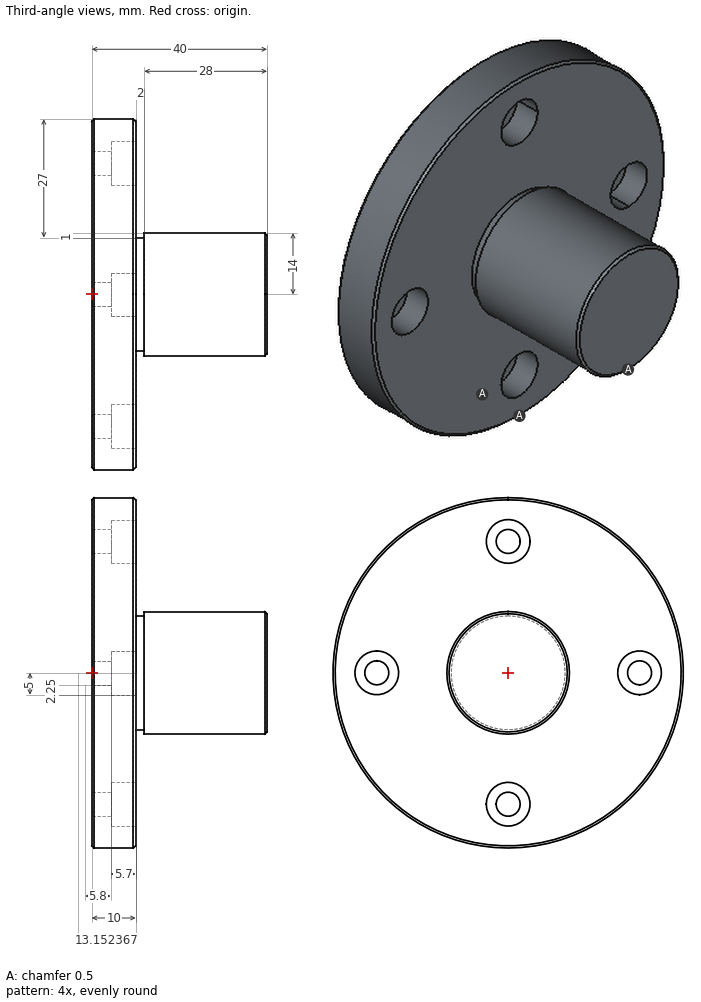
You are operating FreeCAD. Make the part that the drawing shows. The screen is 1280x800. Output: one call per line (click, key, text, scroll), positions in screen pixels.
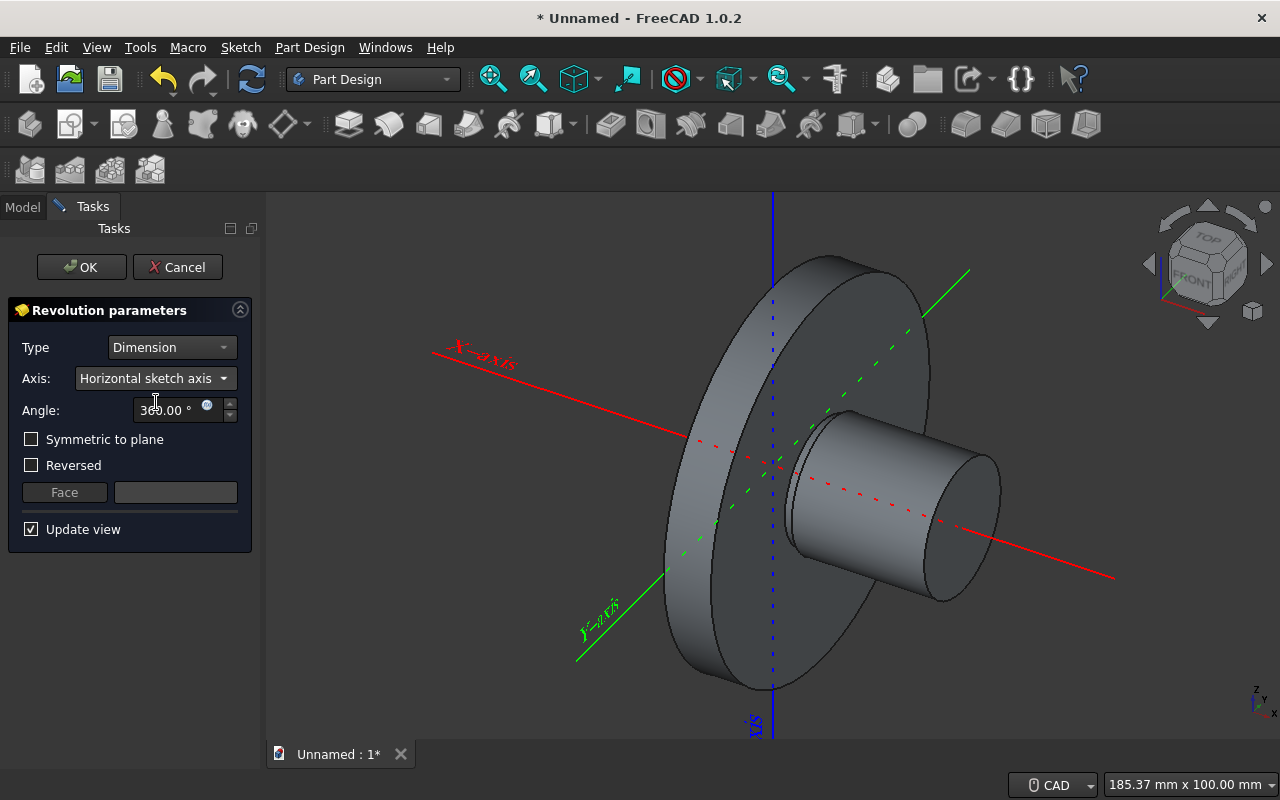
click(82, 267)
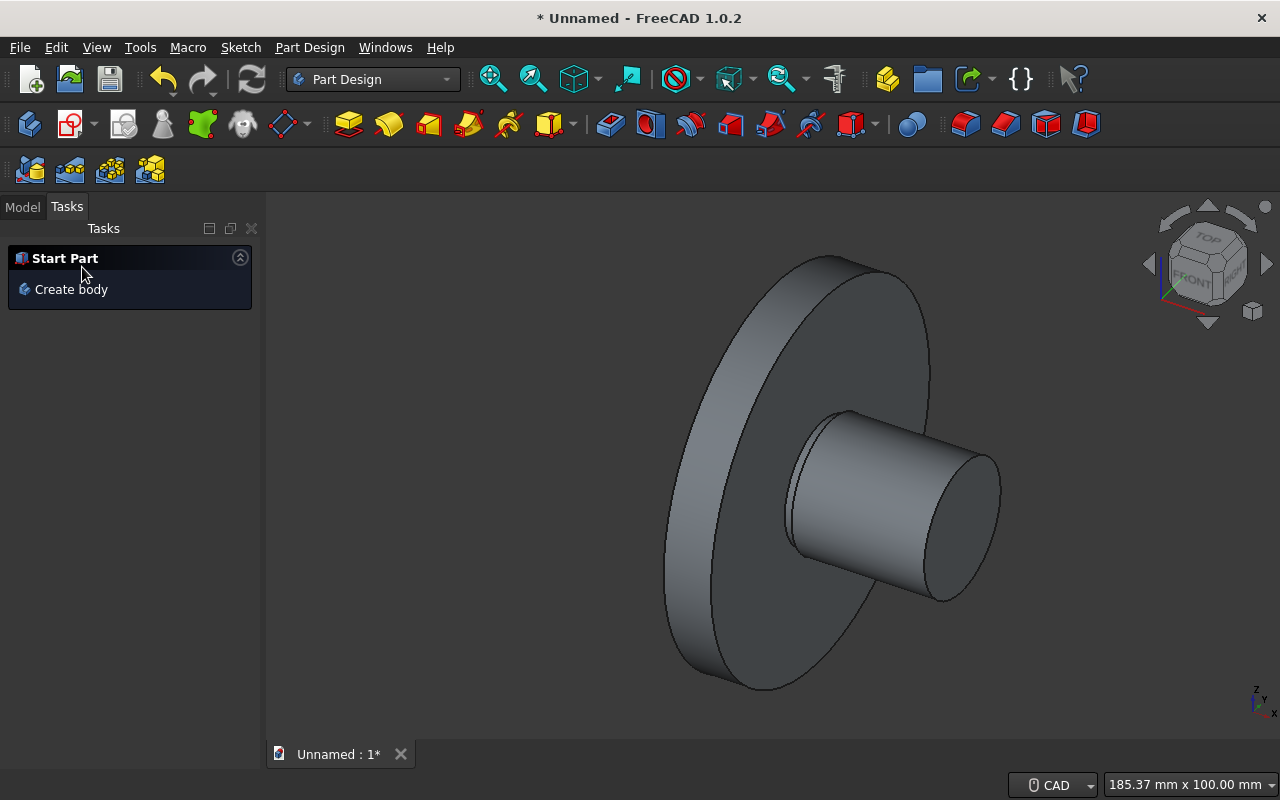
click(494, 80)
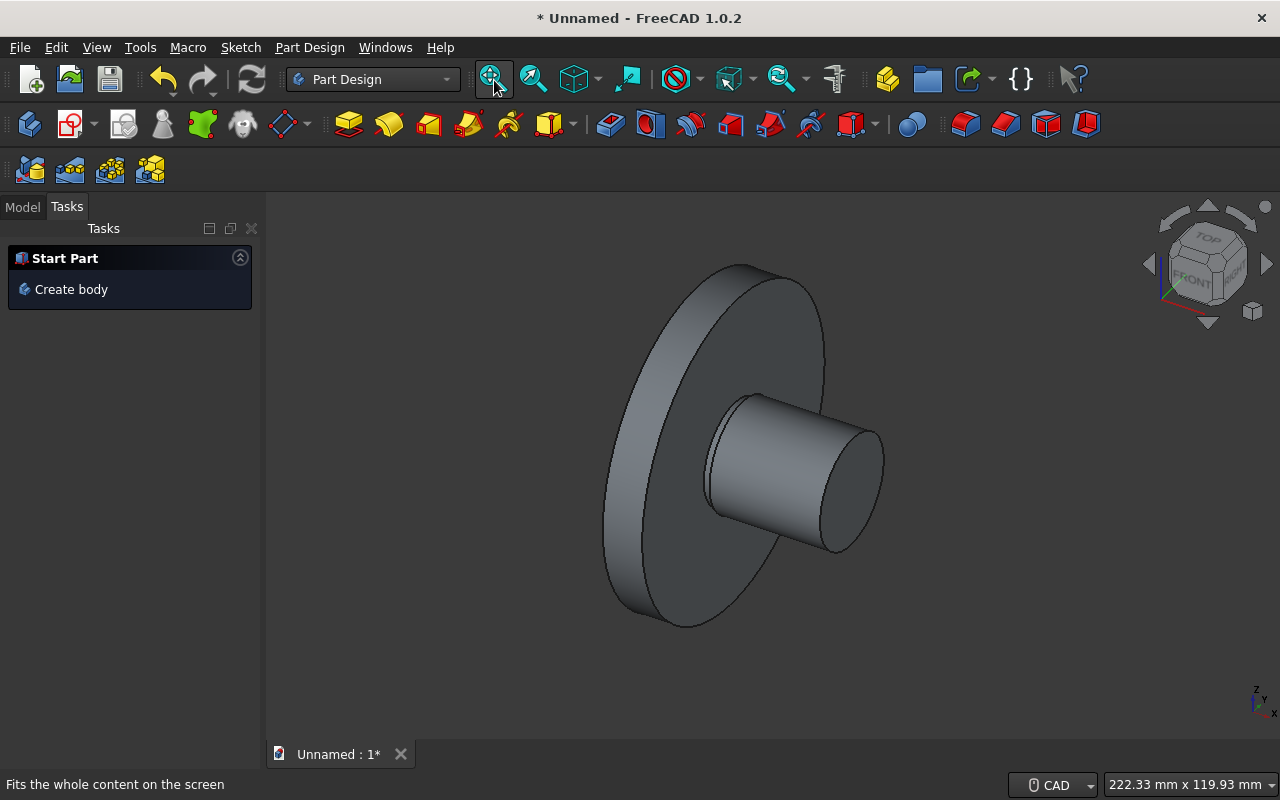
click(820, 522)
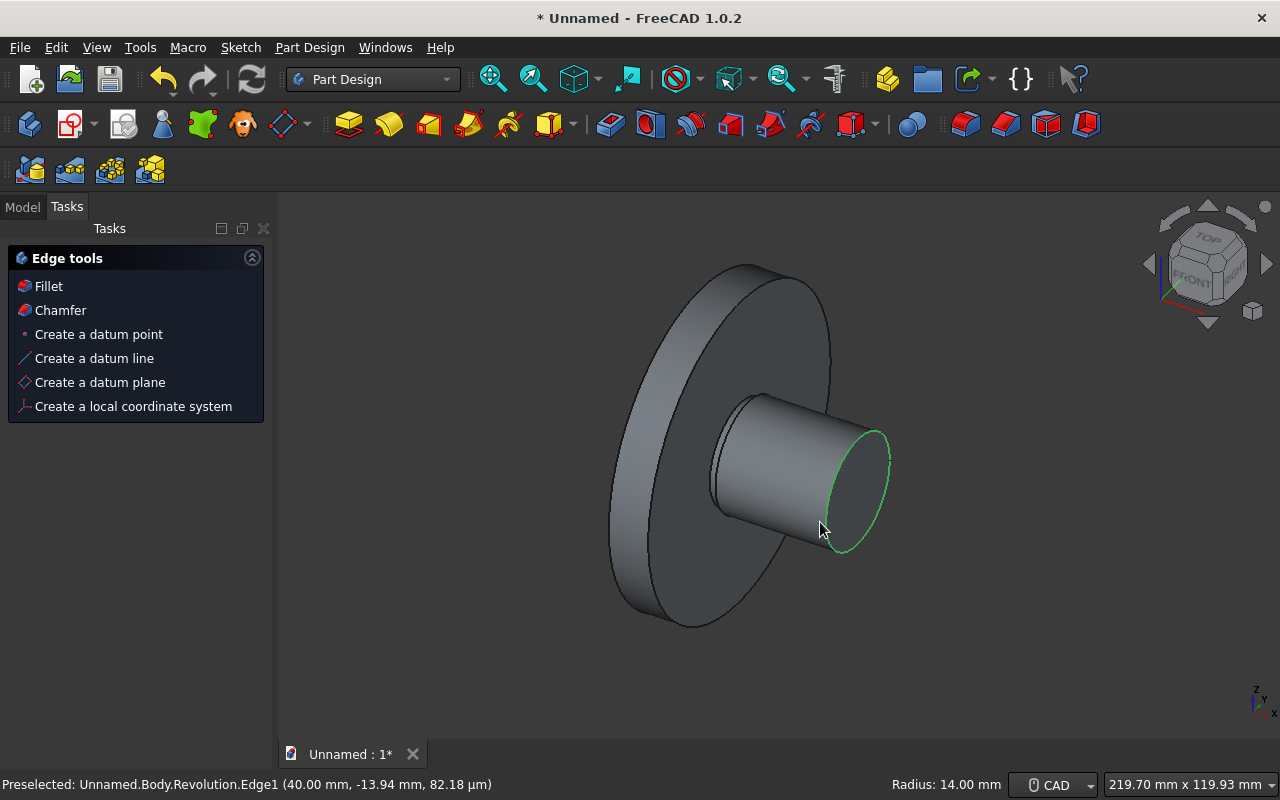
click(648, 542, ctrl)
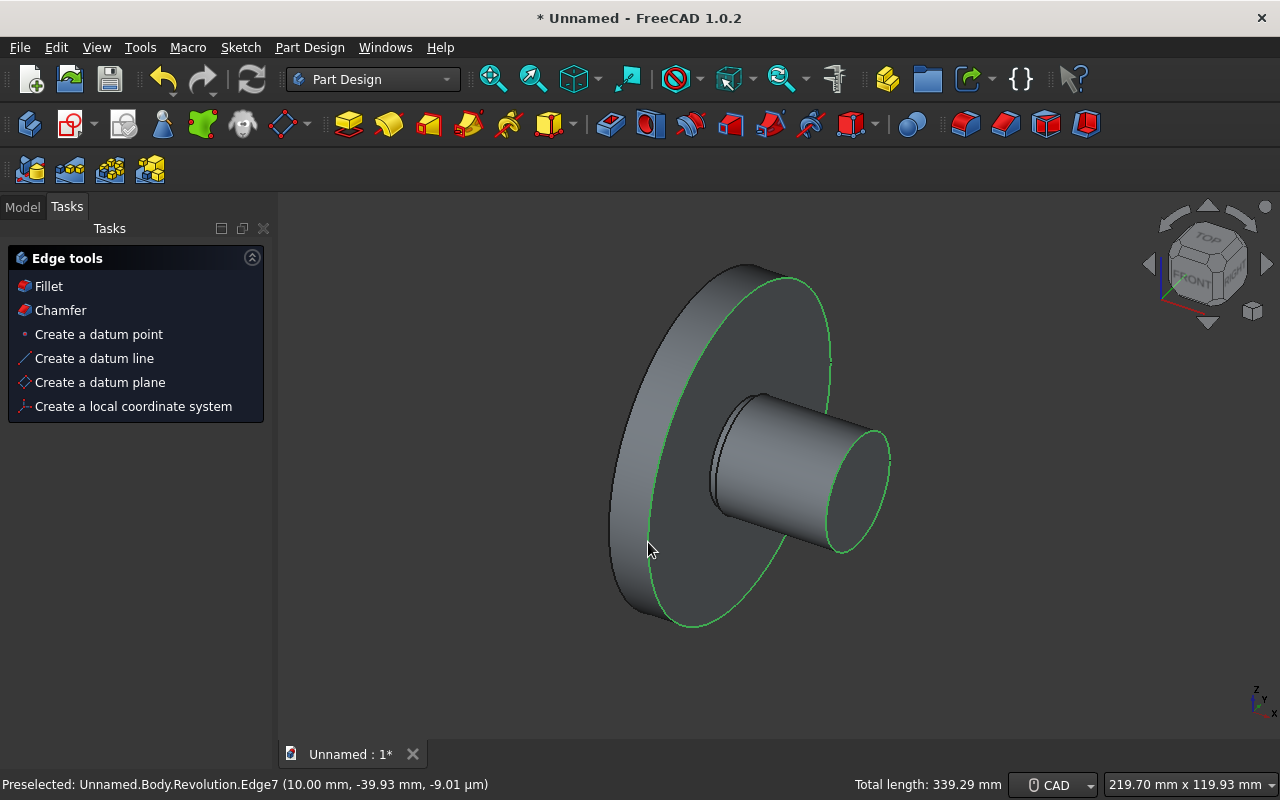
key(0)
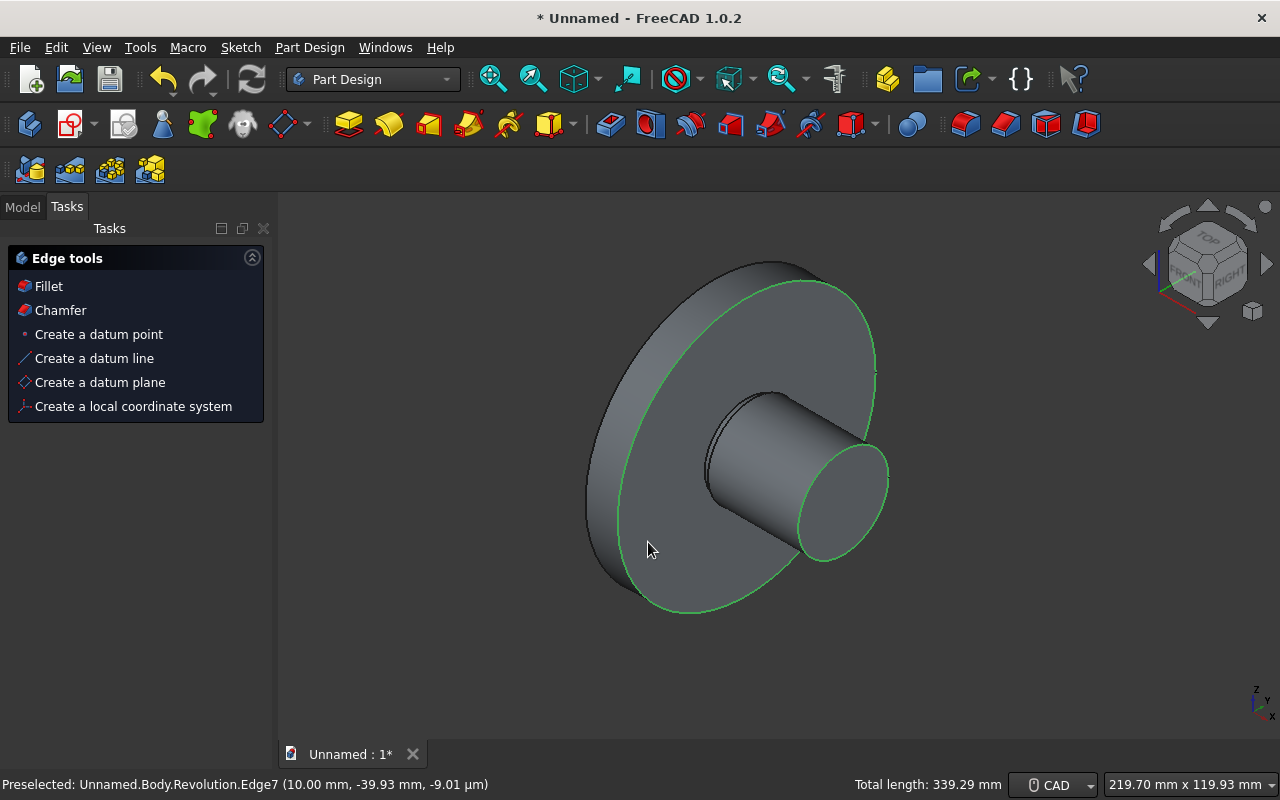
key(2)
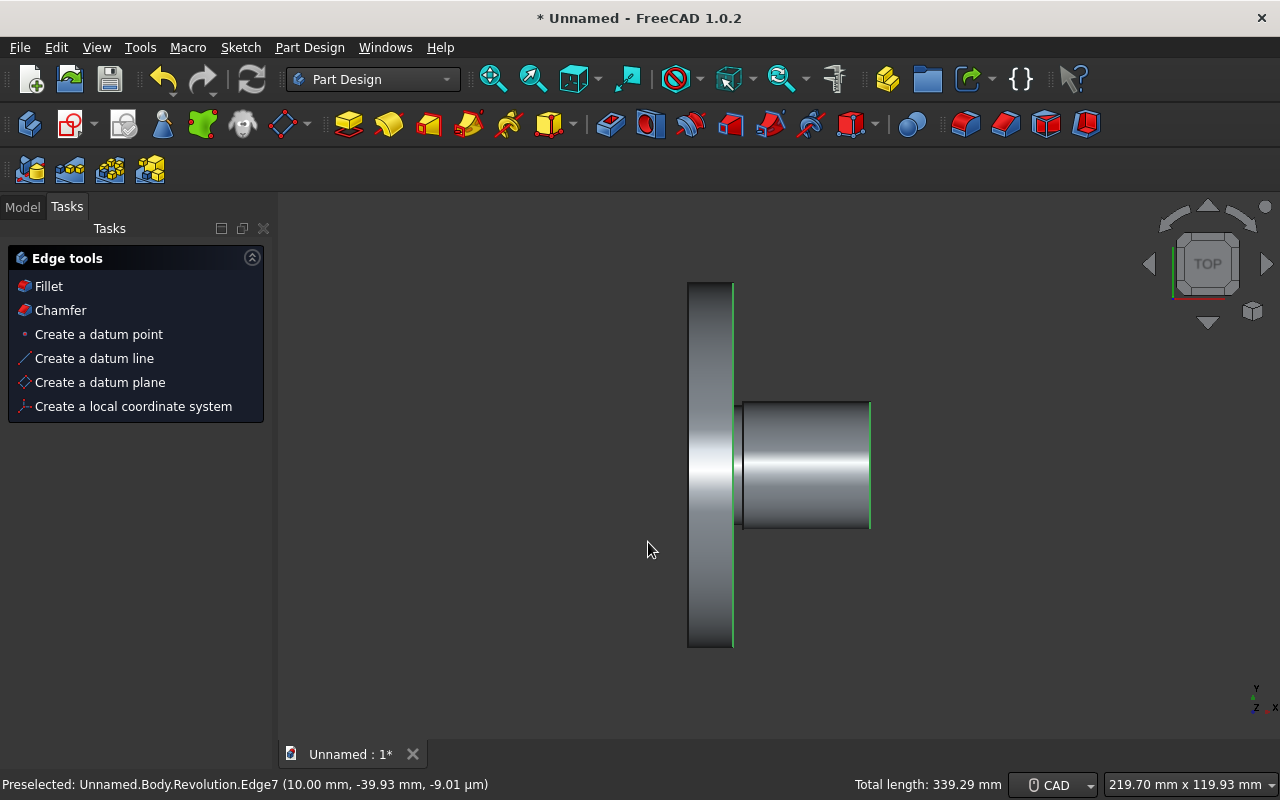
click(688, 612, ctrl)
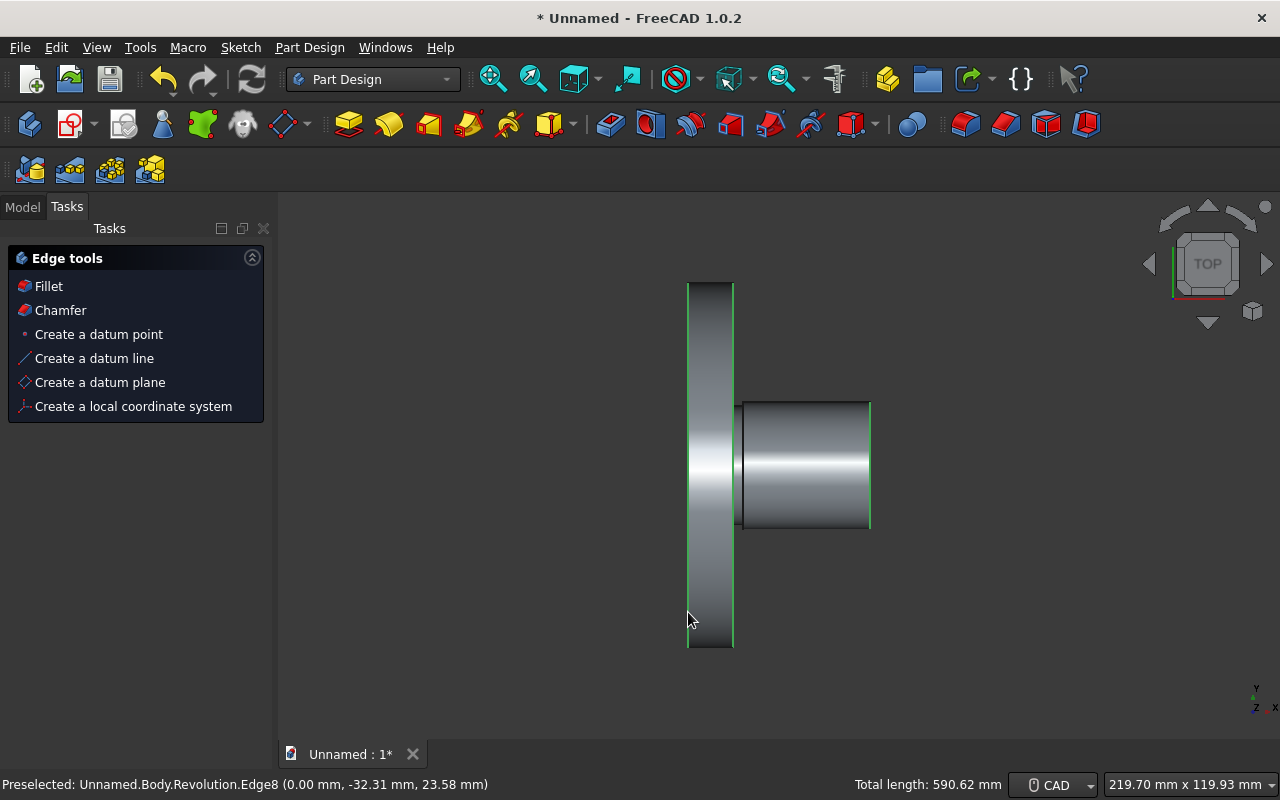
click(1006, 124)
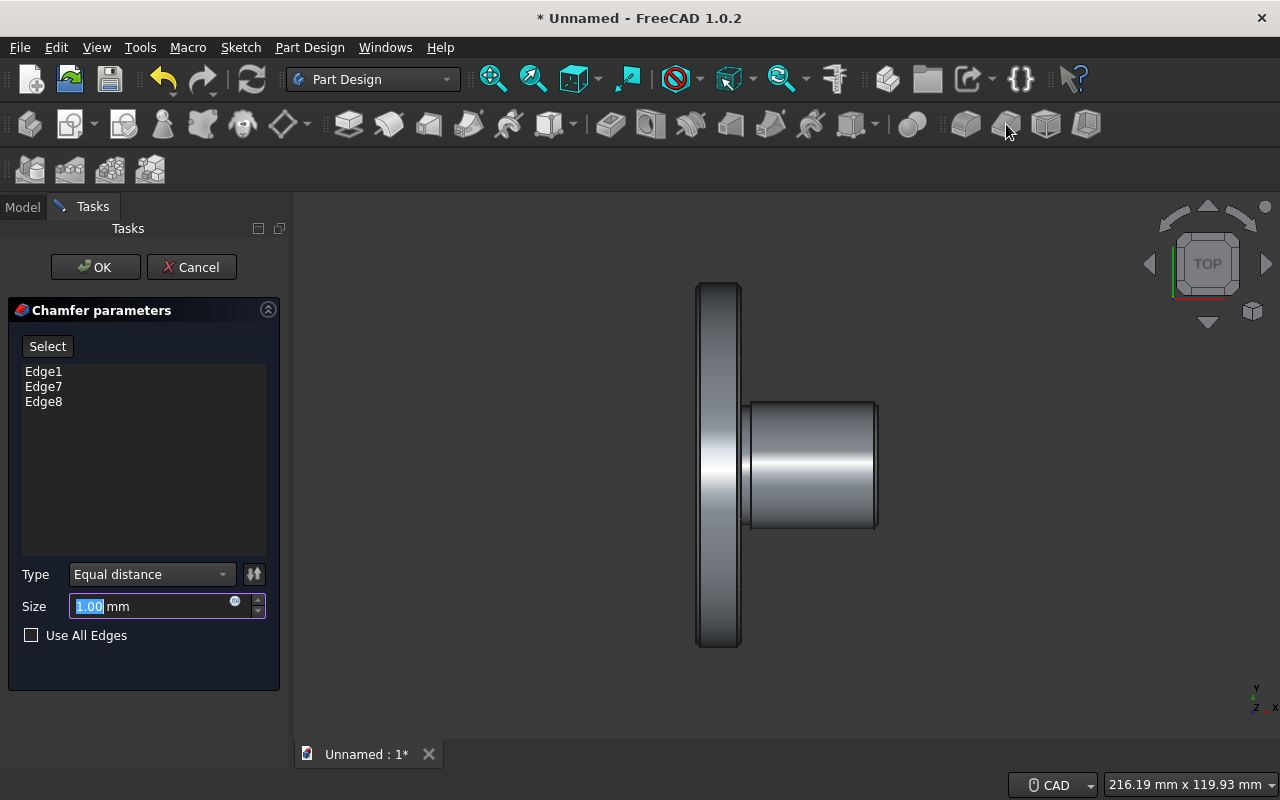
text(0.5)
key(Tab)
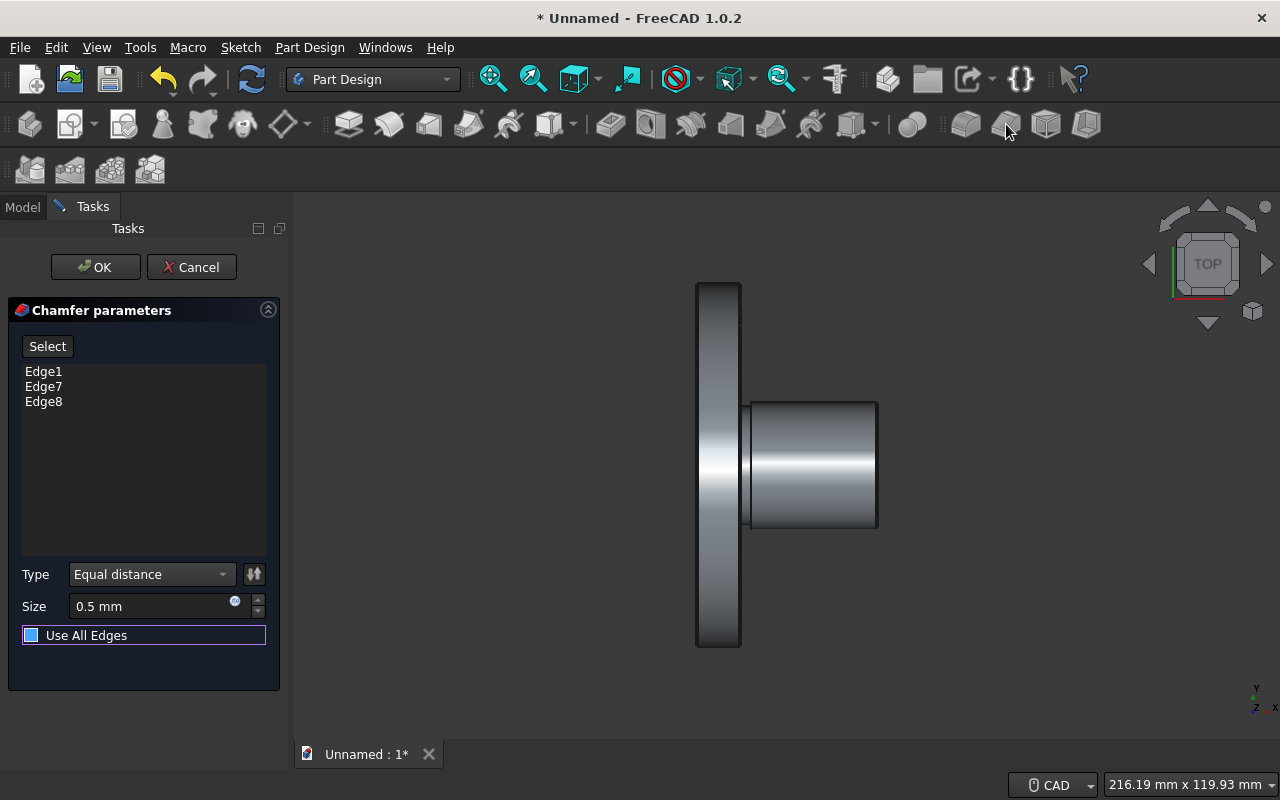
click(96, 267)